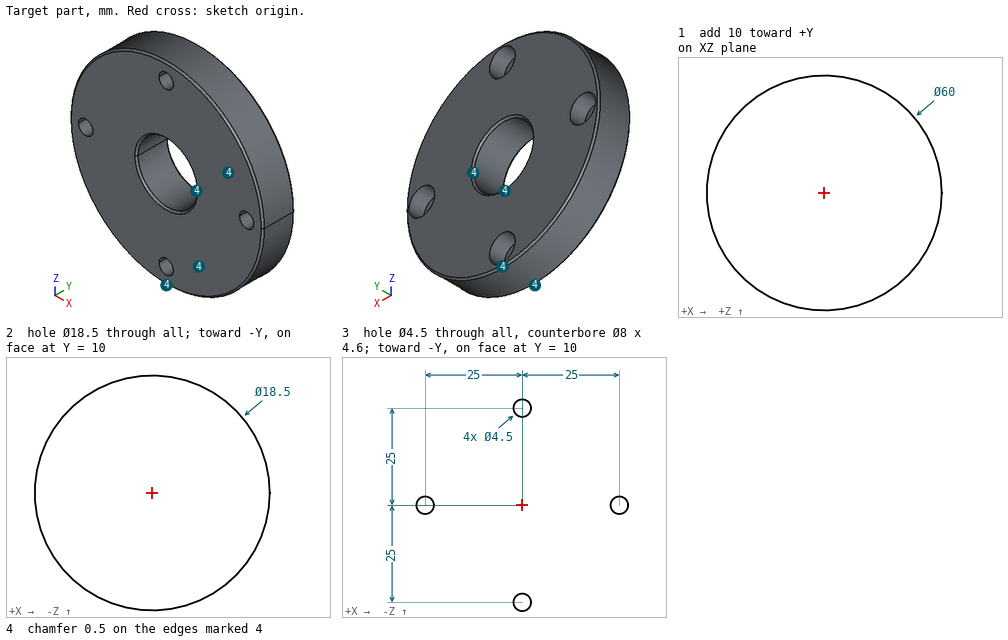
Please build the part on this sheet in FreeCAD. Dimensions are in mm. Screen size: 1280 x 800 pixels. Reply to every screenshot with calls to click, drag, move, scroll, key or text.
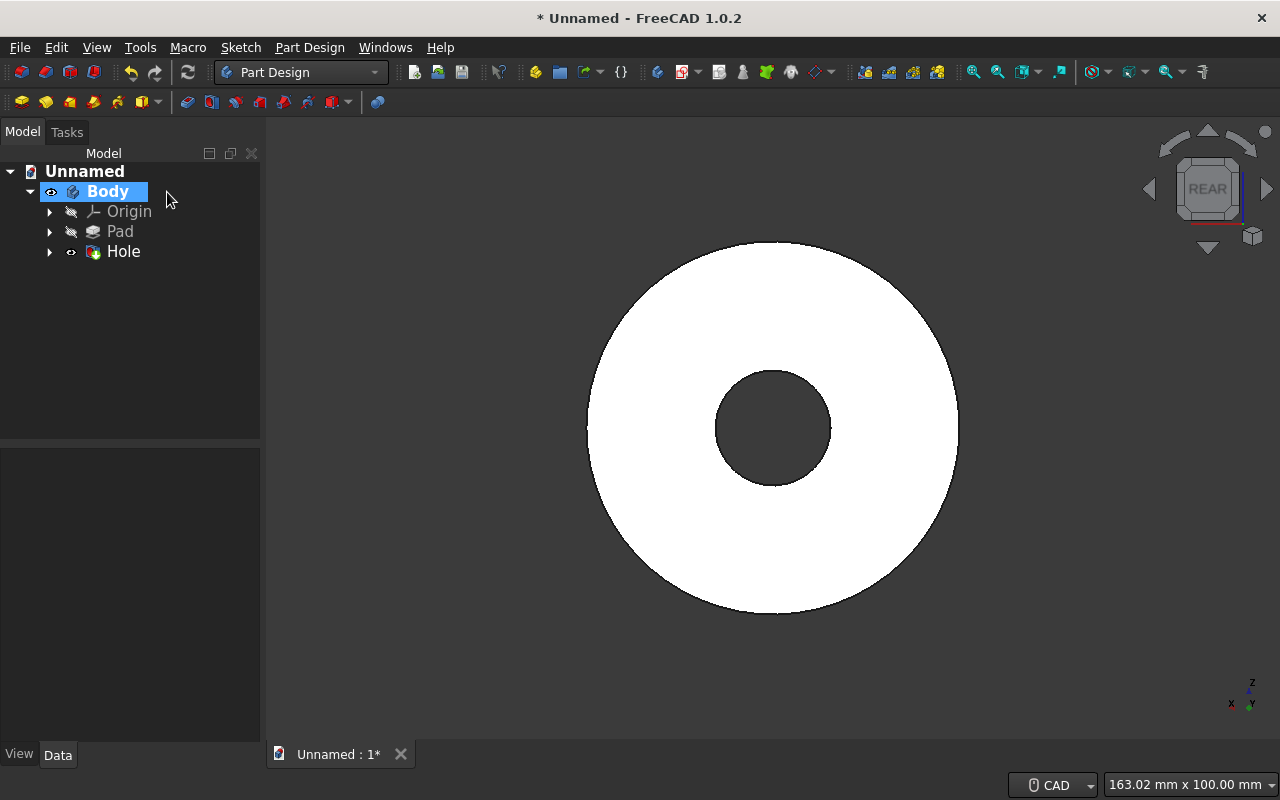
click(666, 480)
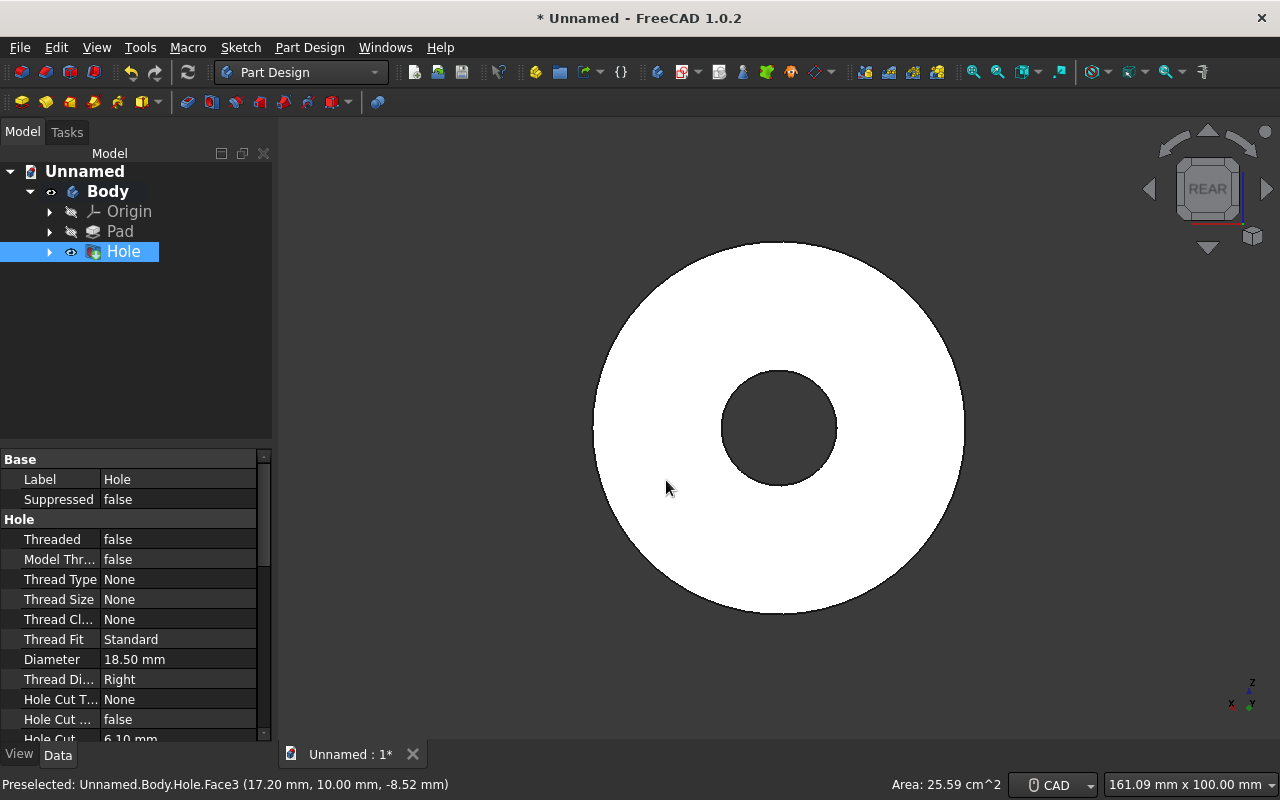
click(682, 72)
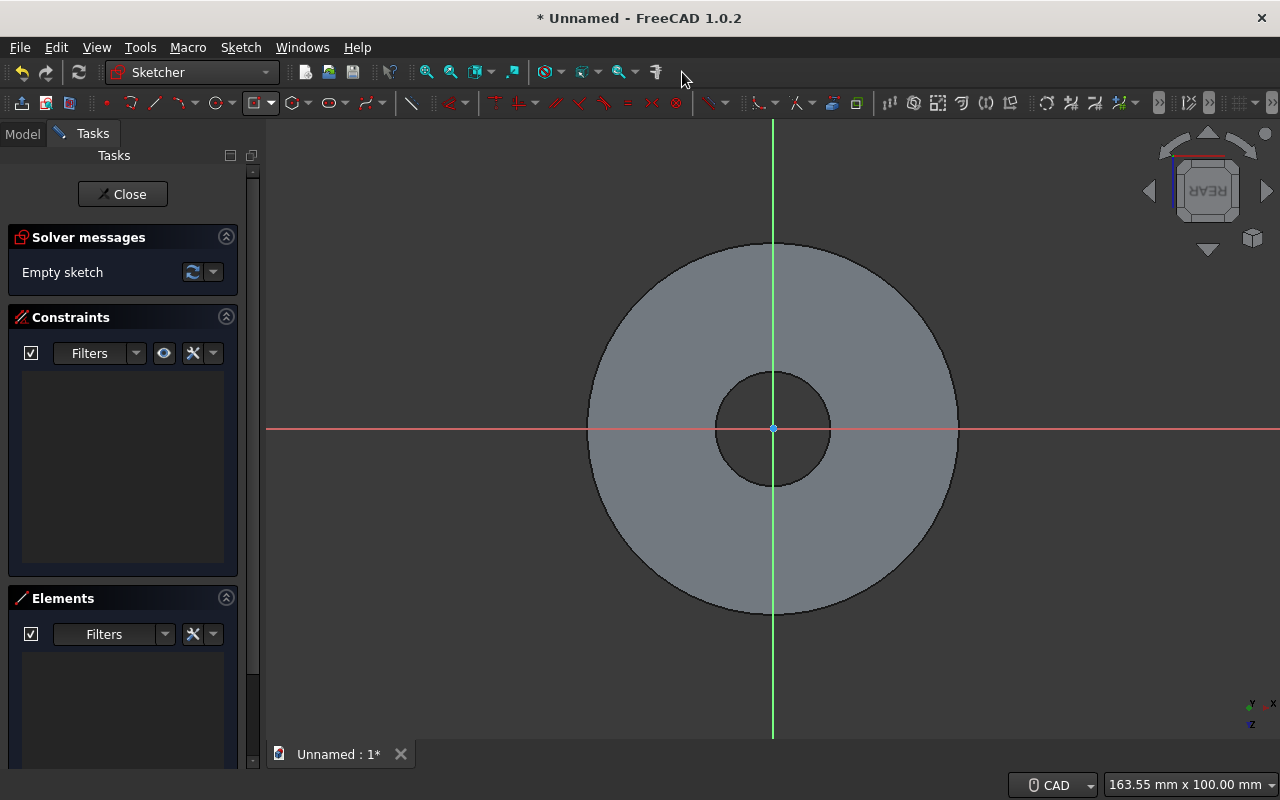
click(216, 104)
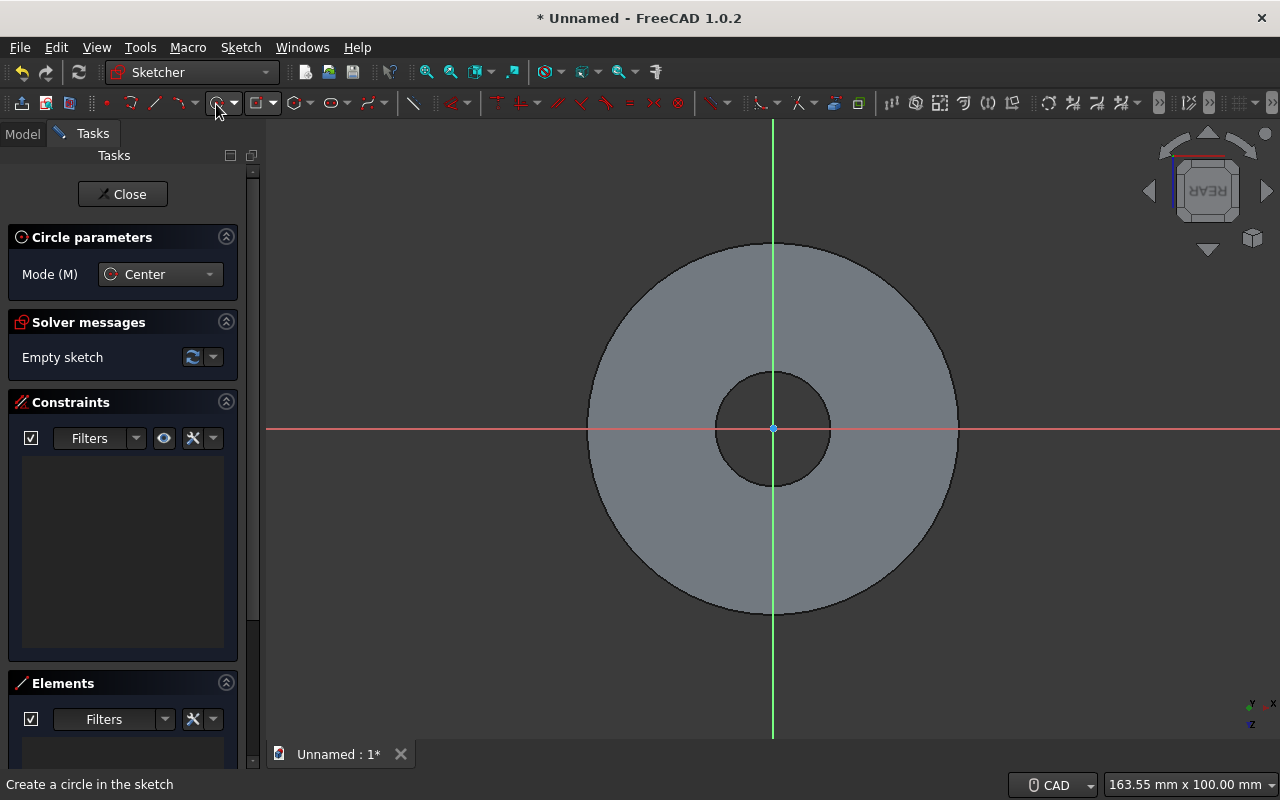
scroll(773, 274, up, 3)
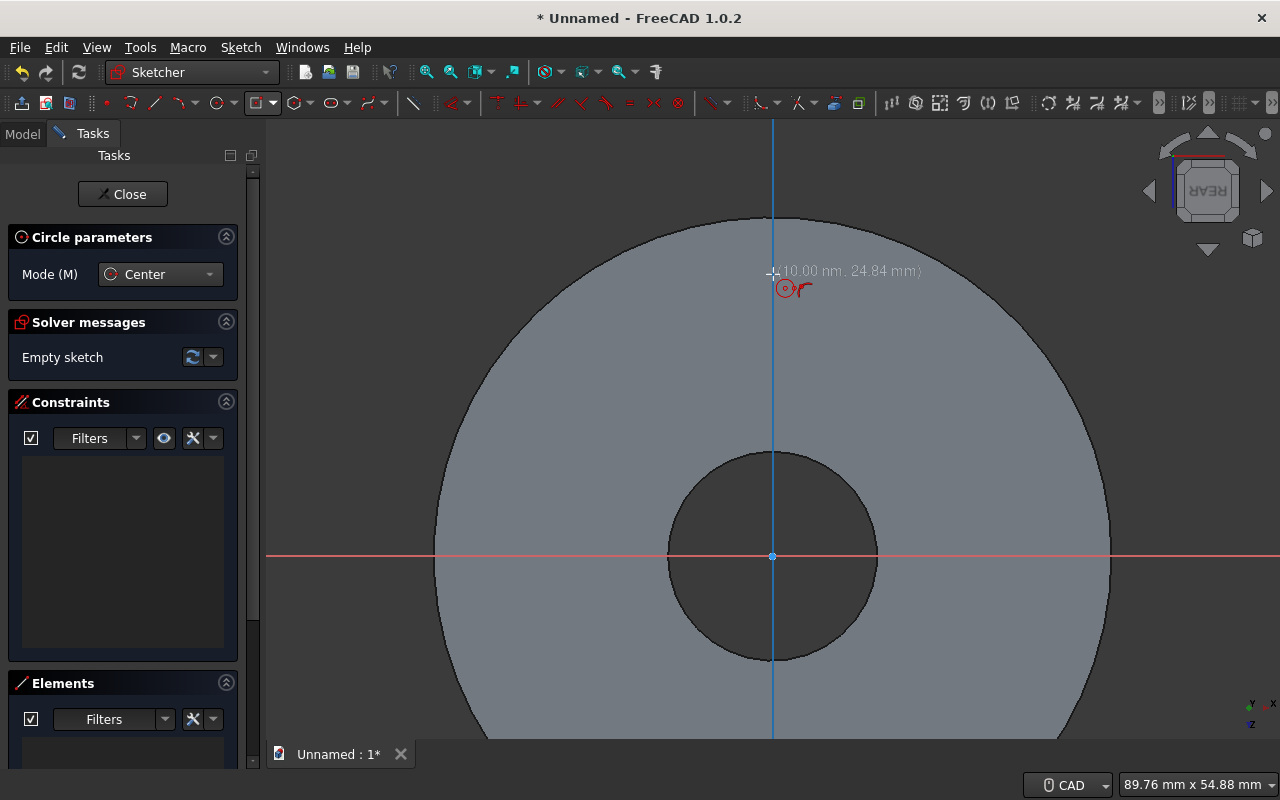
click(773, 274)
click(791, 256)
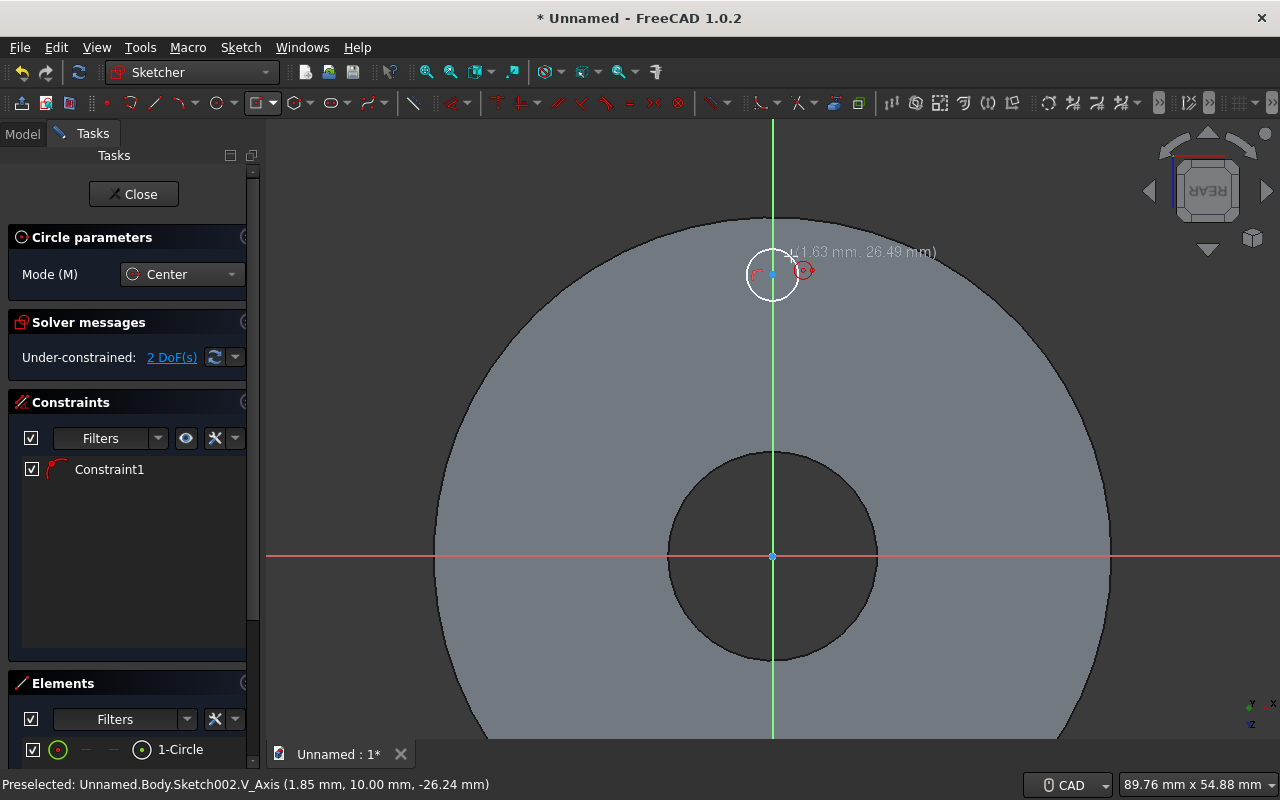
click(1055, 556)
click(1073, 538)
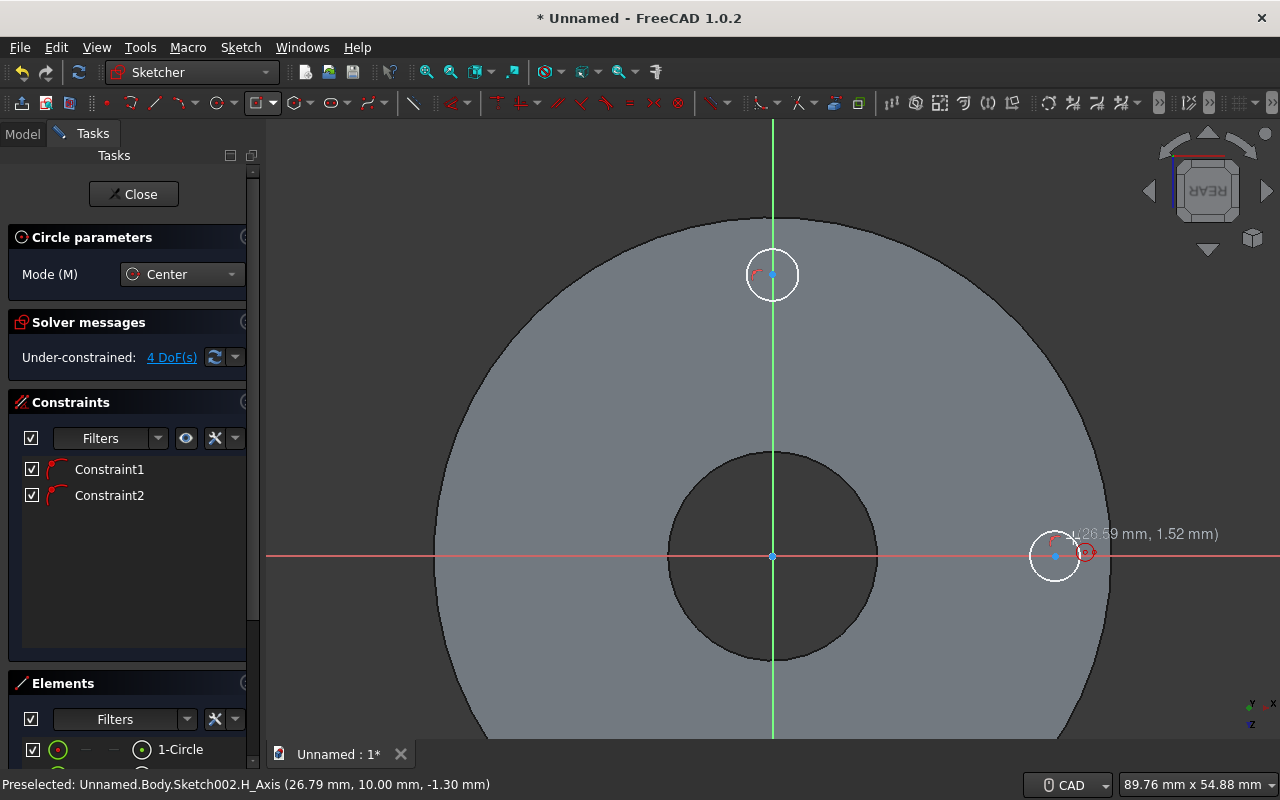
scroll(566, 170, down, 2)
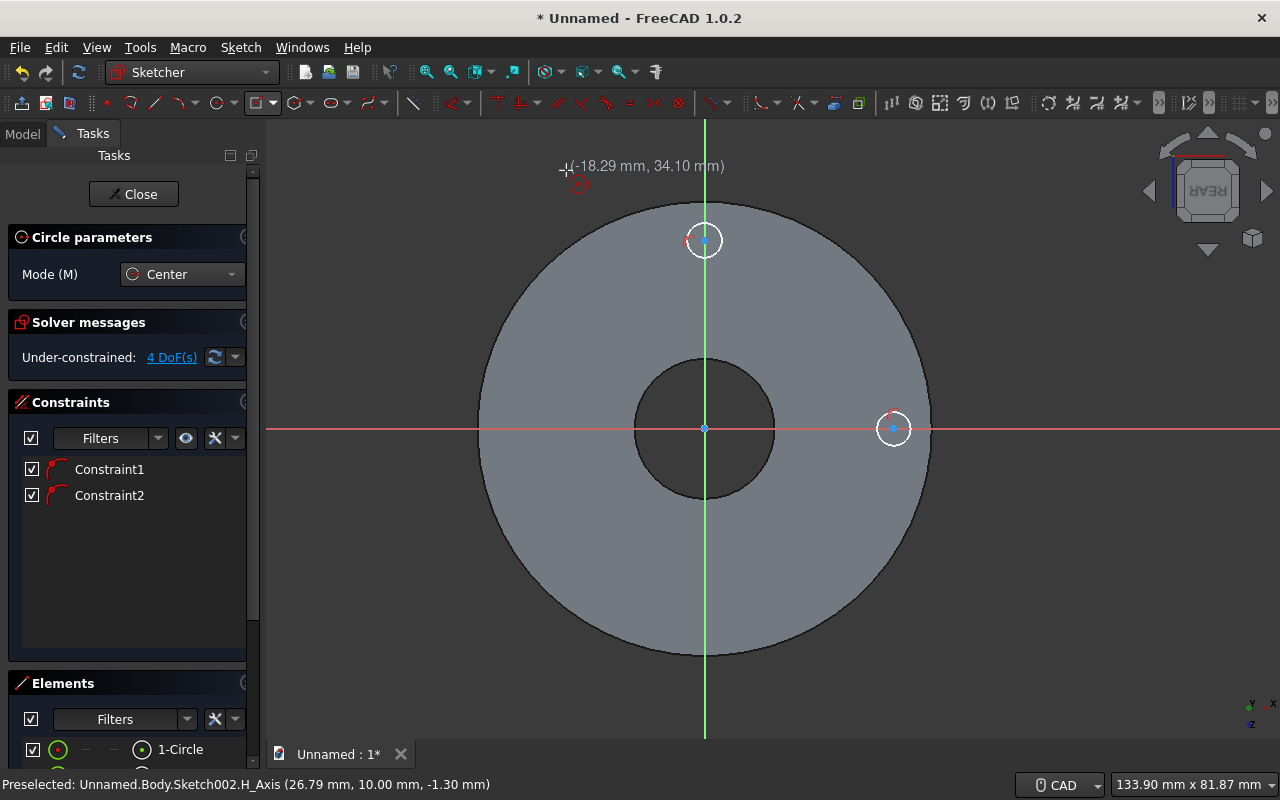
scroll(705, 618, up, 2)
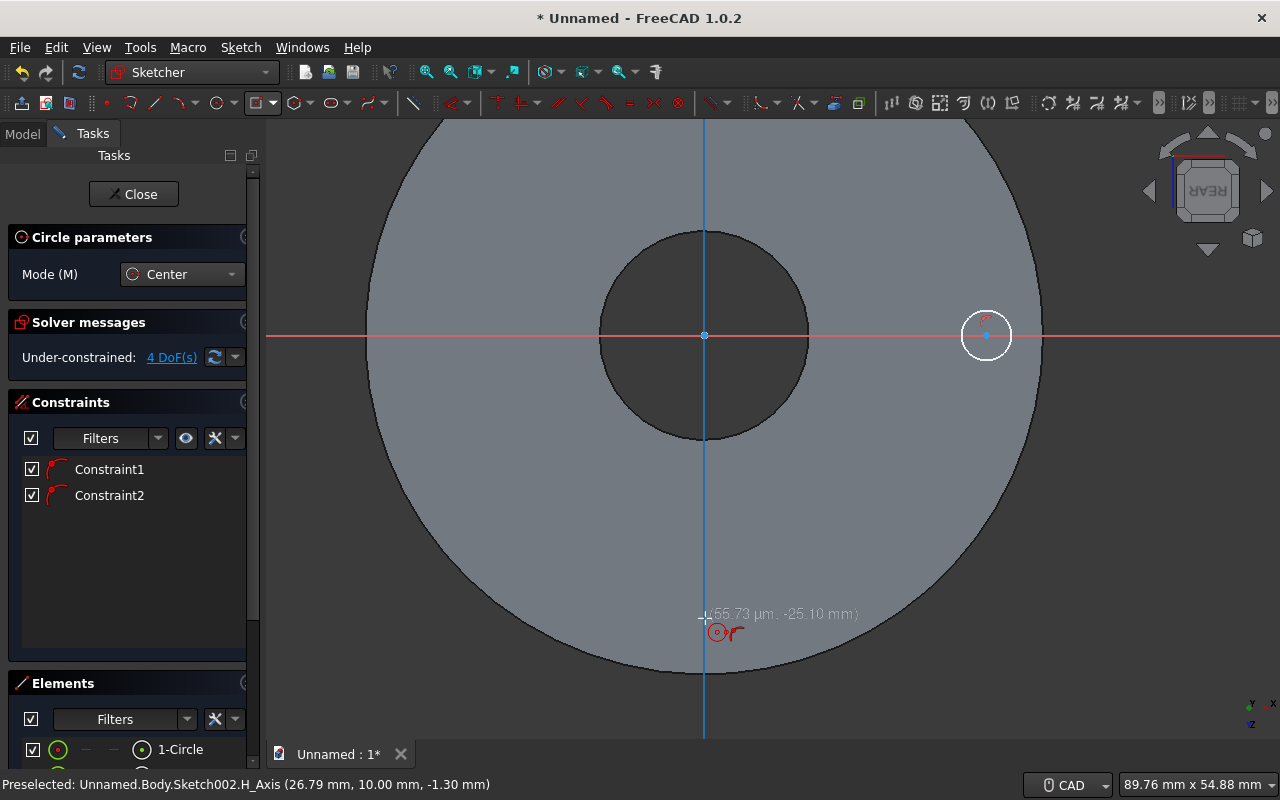
click(704, 618)
click(722, 600)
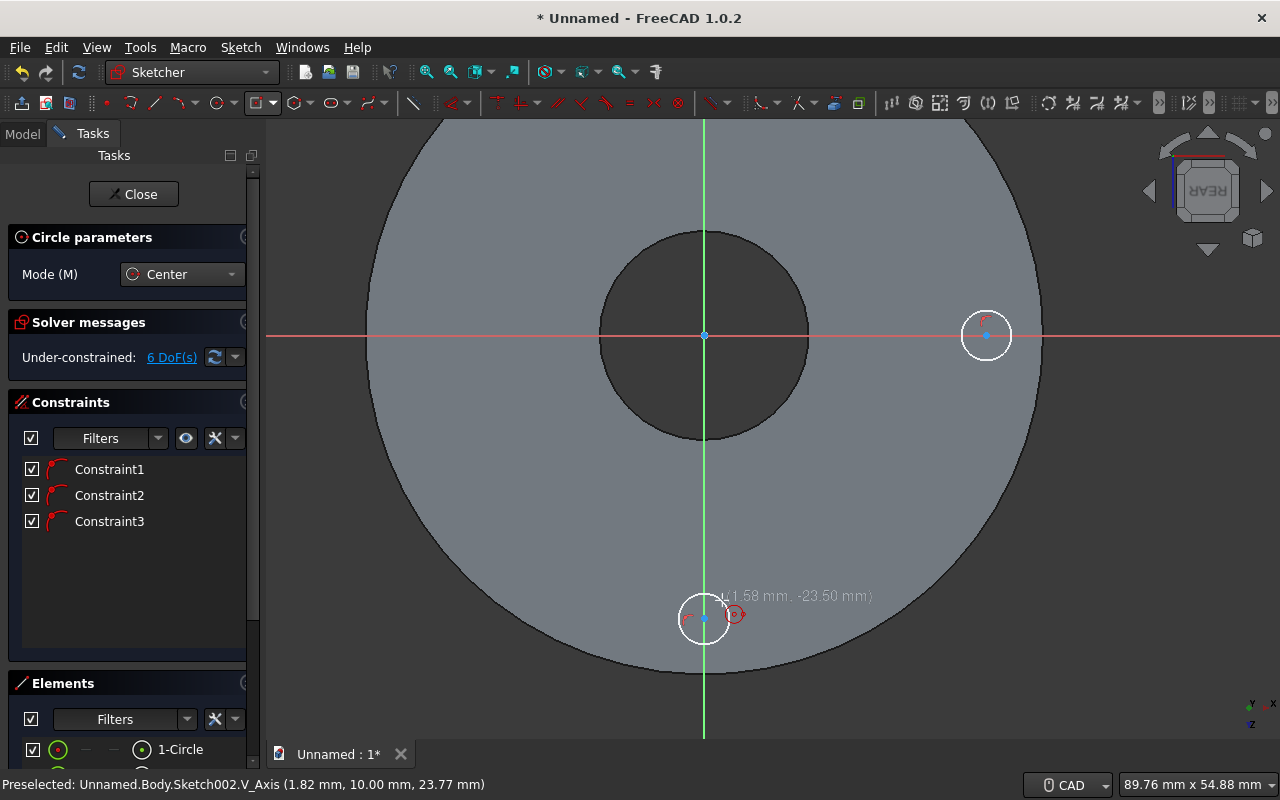
click(422, 336)
click(440, 318)
key(Escape)